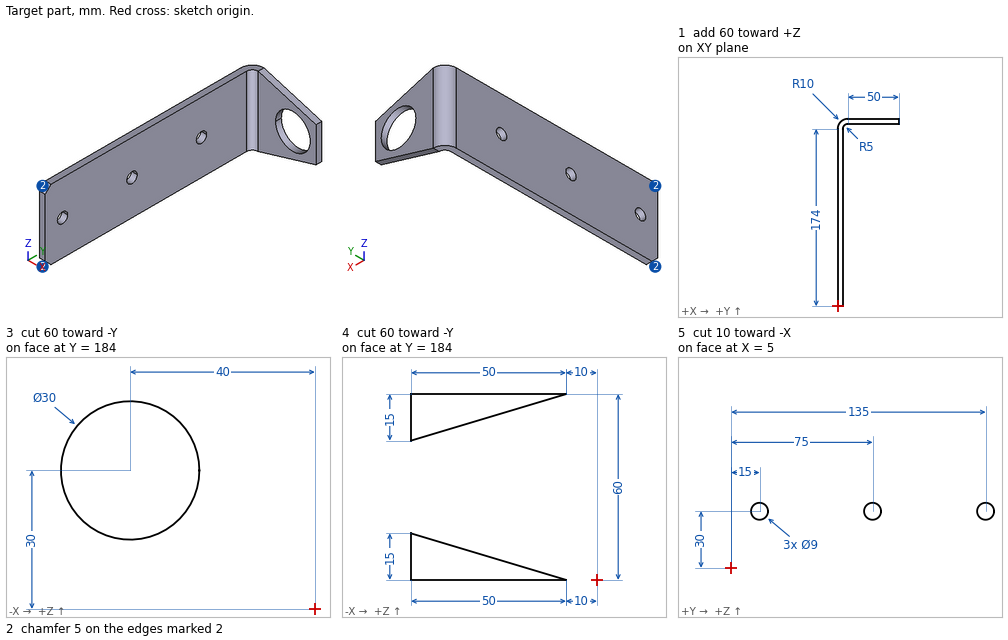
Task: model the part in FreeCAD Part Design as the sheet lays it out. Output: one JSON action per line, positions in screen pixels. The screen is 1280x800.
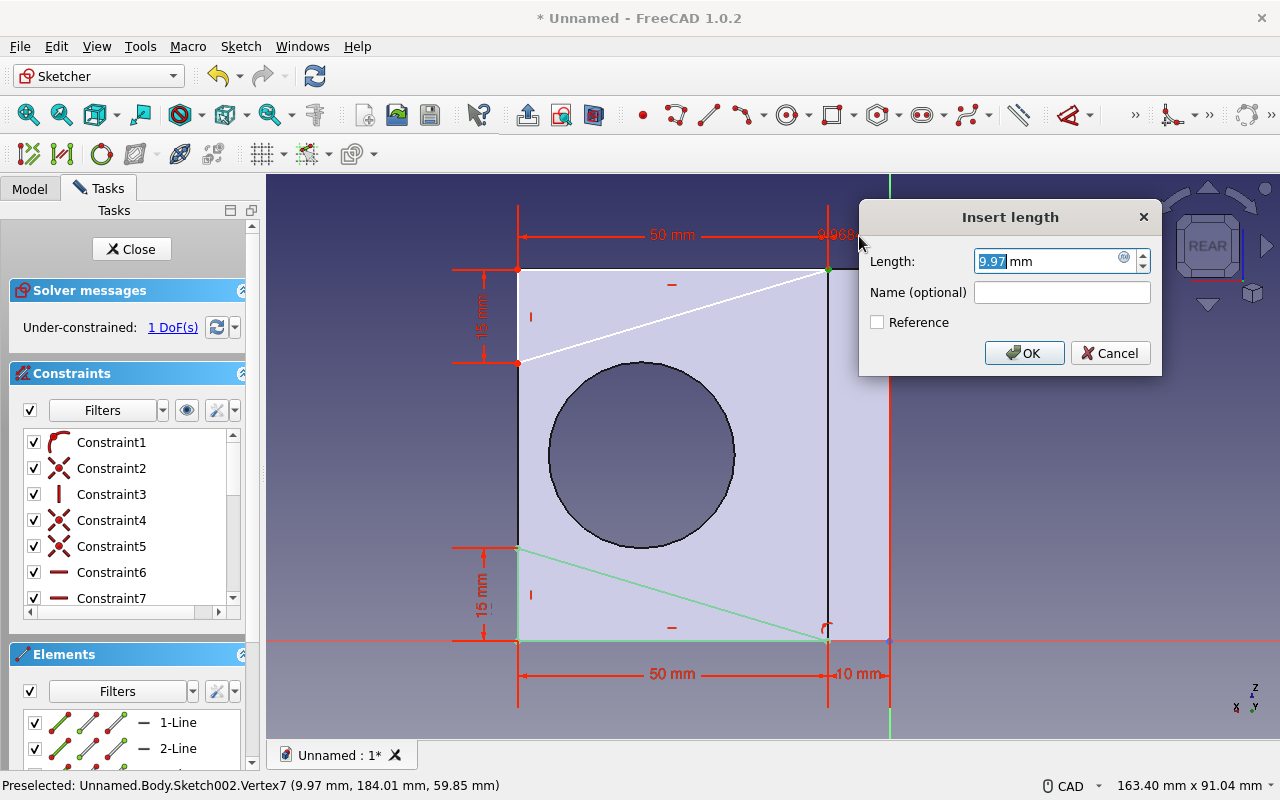
{"action": "type", "text": "10"}
{"action": "key", "text": "Return"}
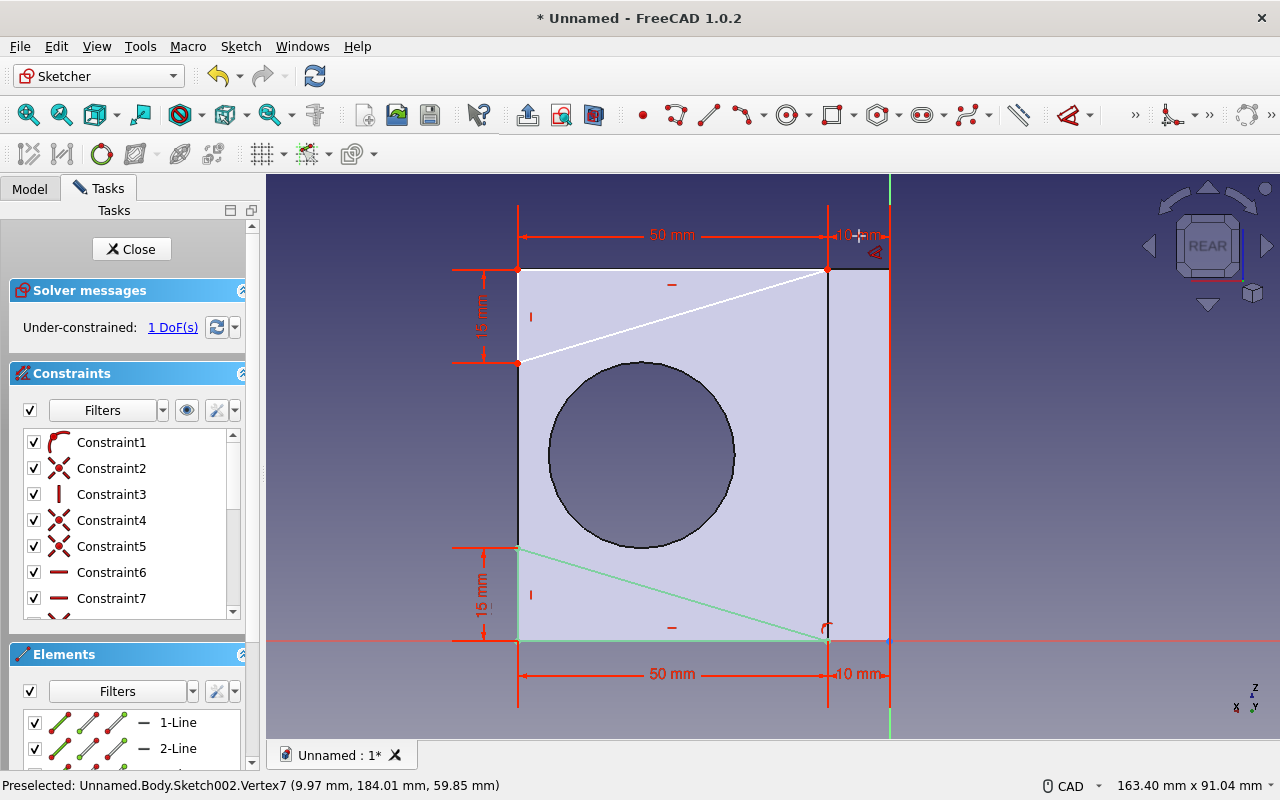
{"action": "left_click", "coordinate": [828, 270]}
{"action": "left_click", "coordinate": [924, 456]}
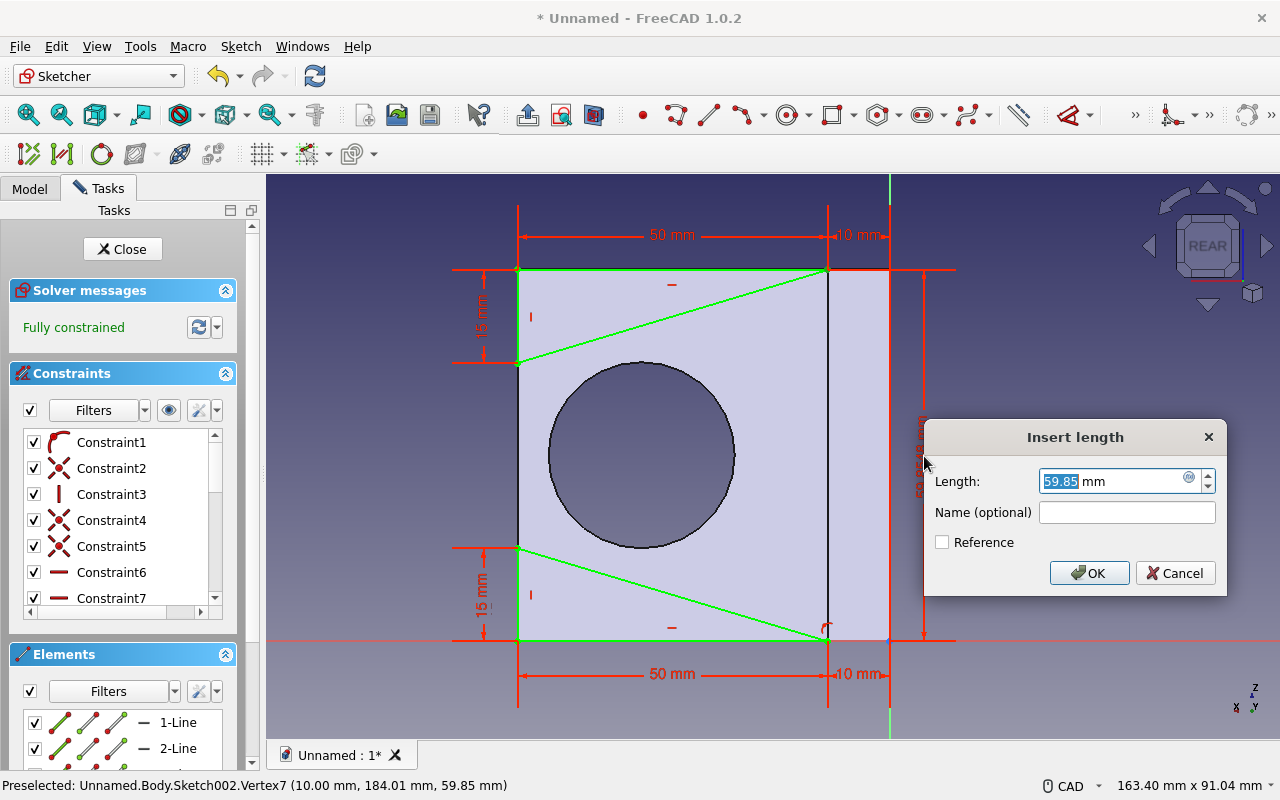
{"action": "type", "text": "60"}
{"action": "key", "text": "Return"}
{"action": "key", "text": "Escape"}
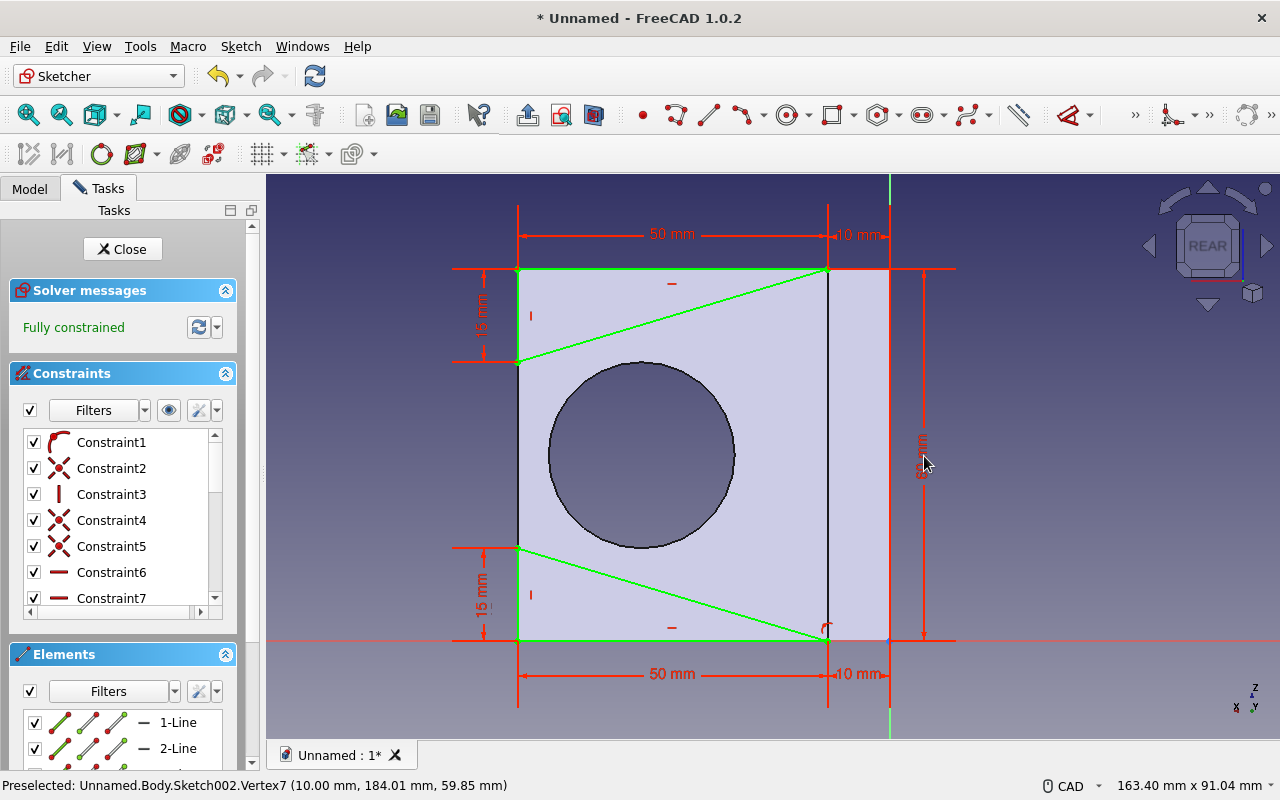
{"action": "left_click", "coordinate": [123, 249]}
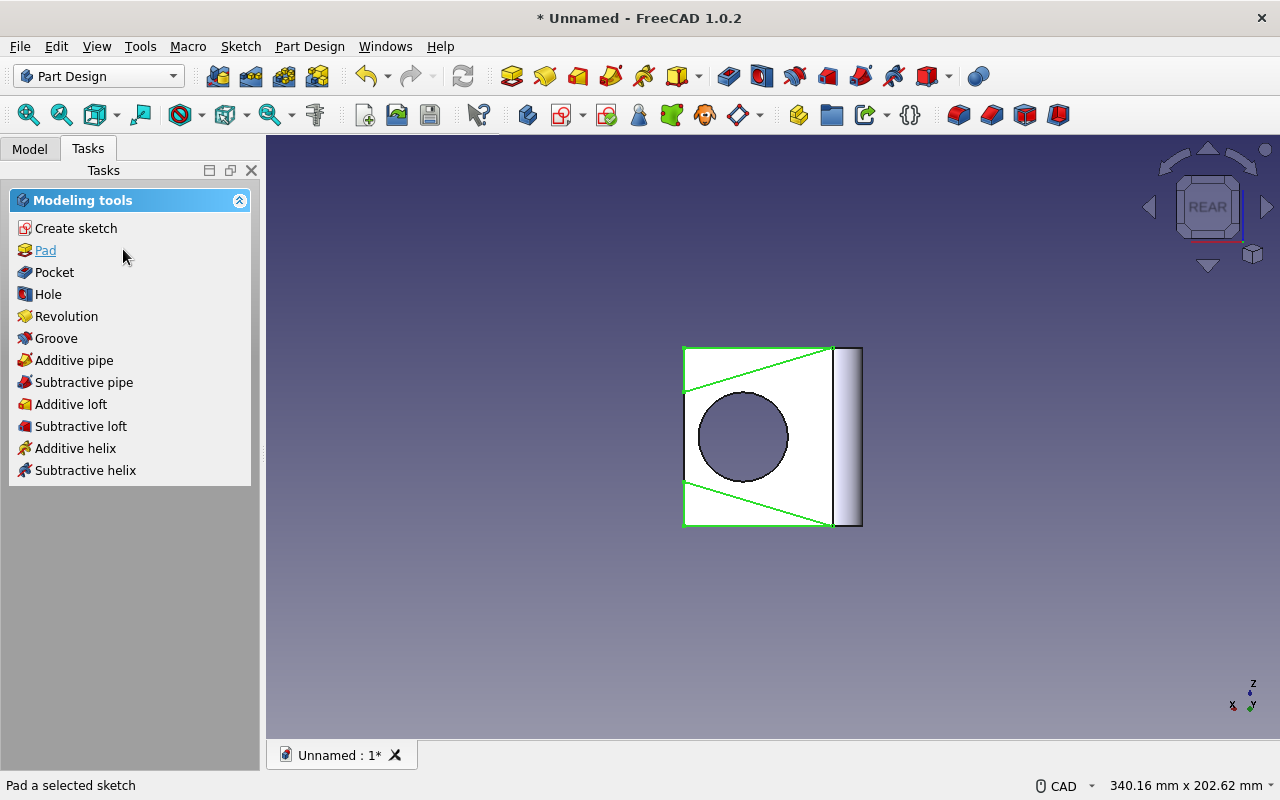
{"action": "left_click", "coordinate": [729, 76]}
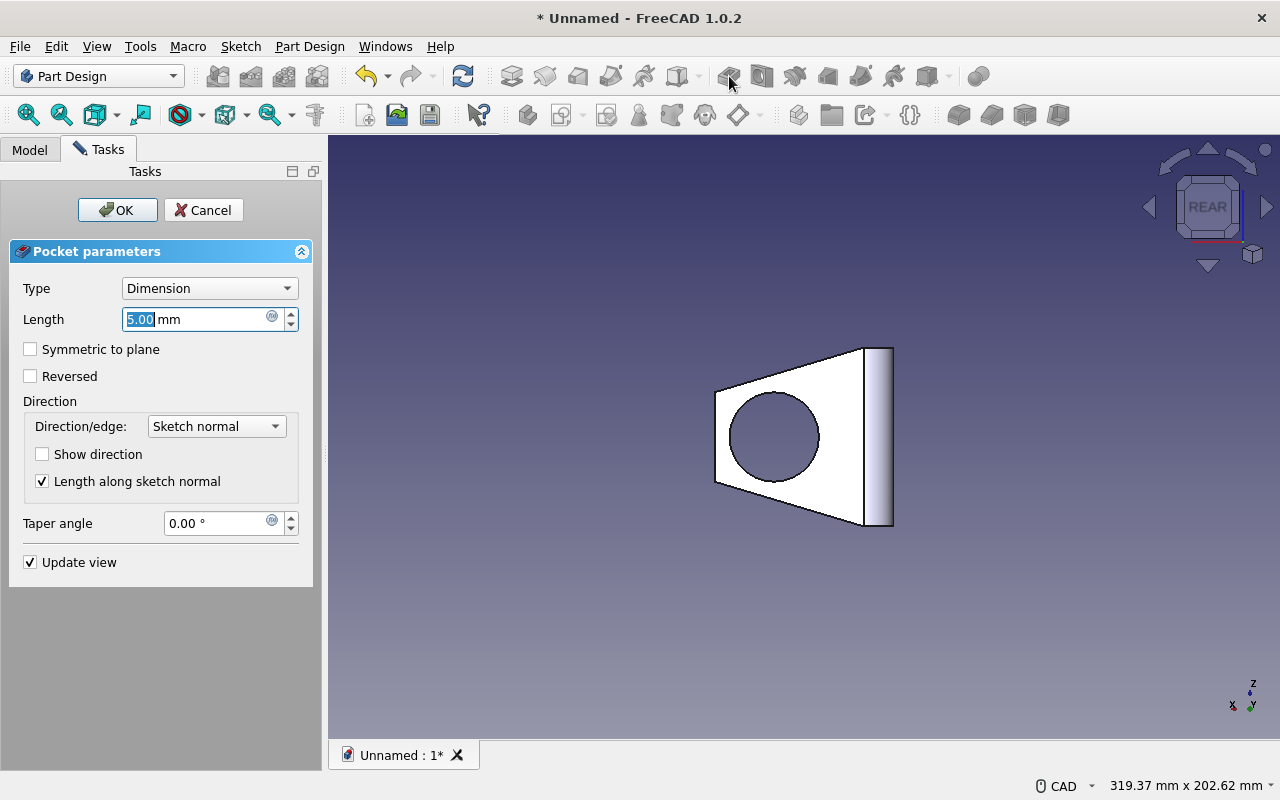
{"action": "type", "text": "60"}
{"action": "key", "text": "Tab"}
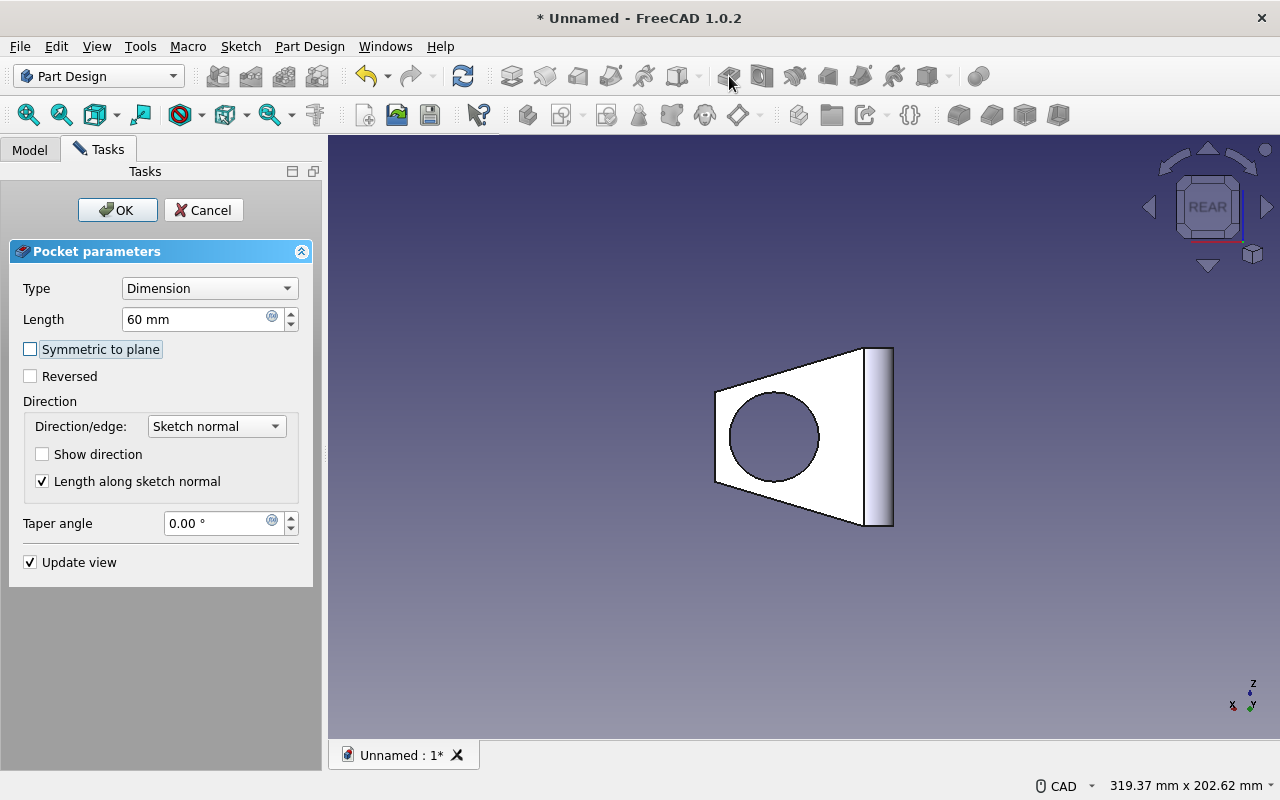
{"action": "left_click", "coordinate": [118, 210]}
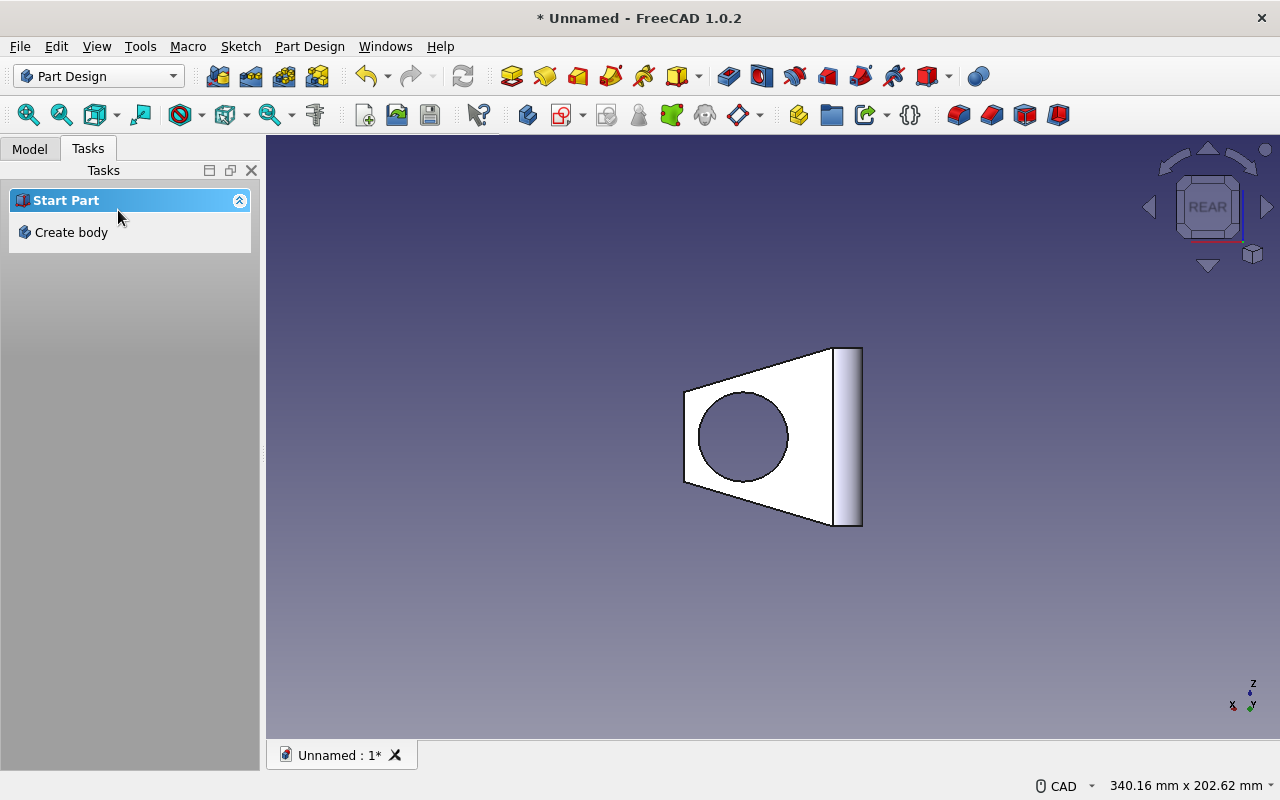
{"action": "key", "text": "v f"}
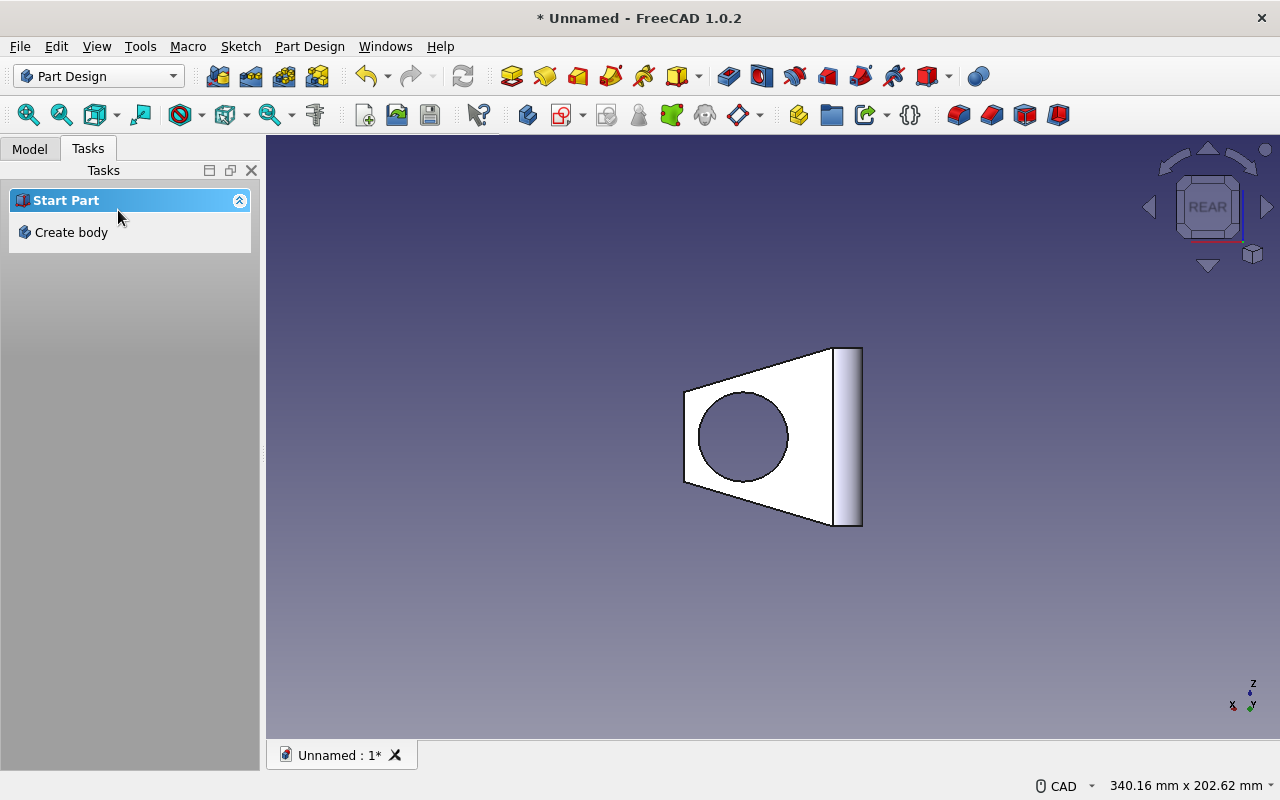
{"action": "key", "text": "0"}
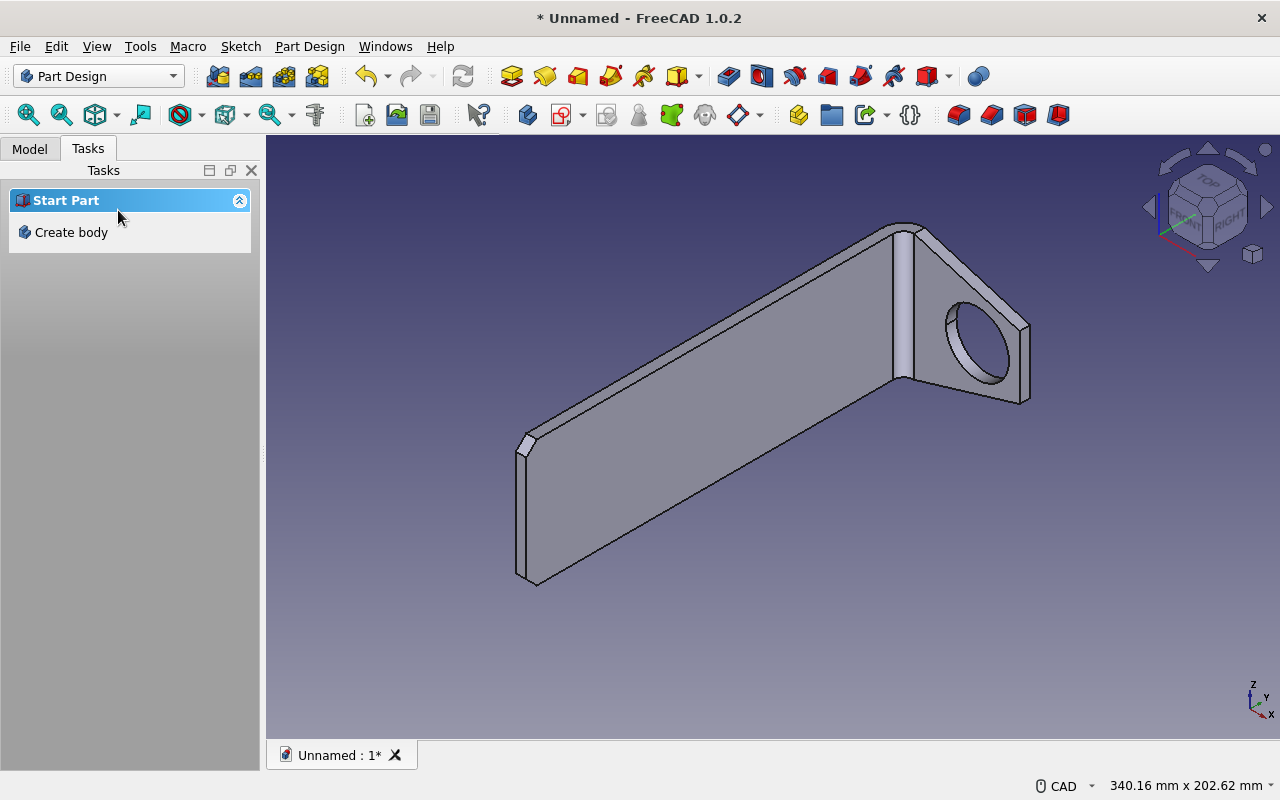
{"action": "left_click", "coordinate": [815, 351]}